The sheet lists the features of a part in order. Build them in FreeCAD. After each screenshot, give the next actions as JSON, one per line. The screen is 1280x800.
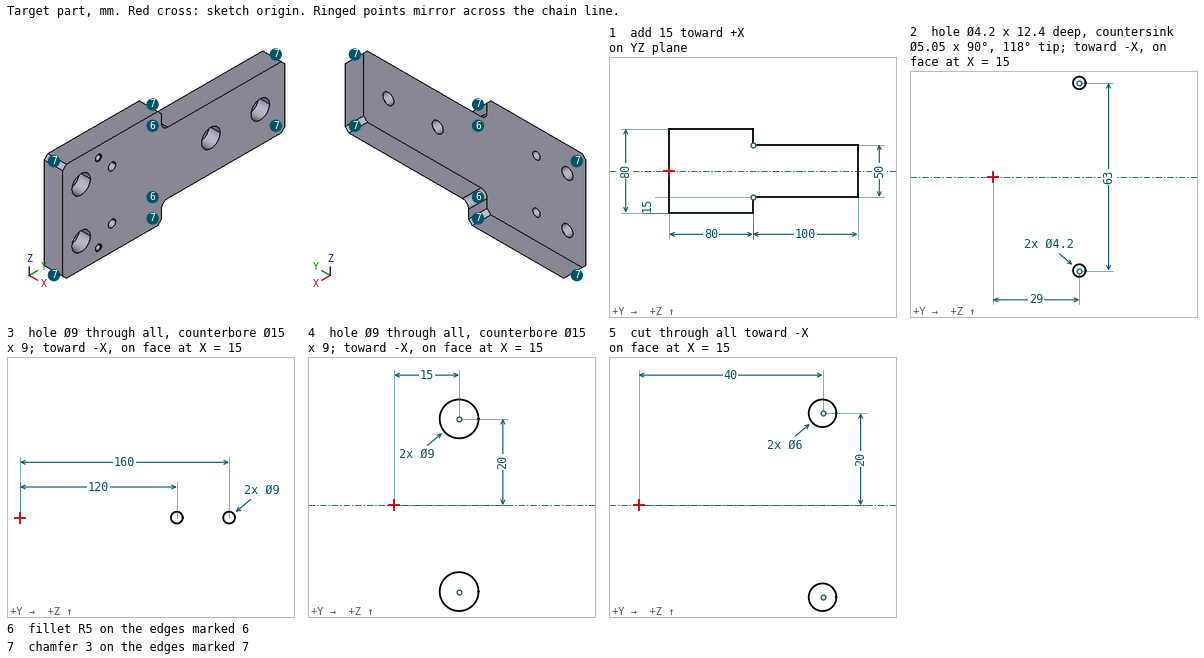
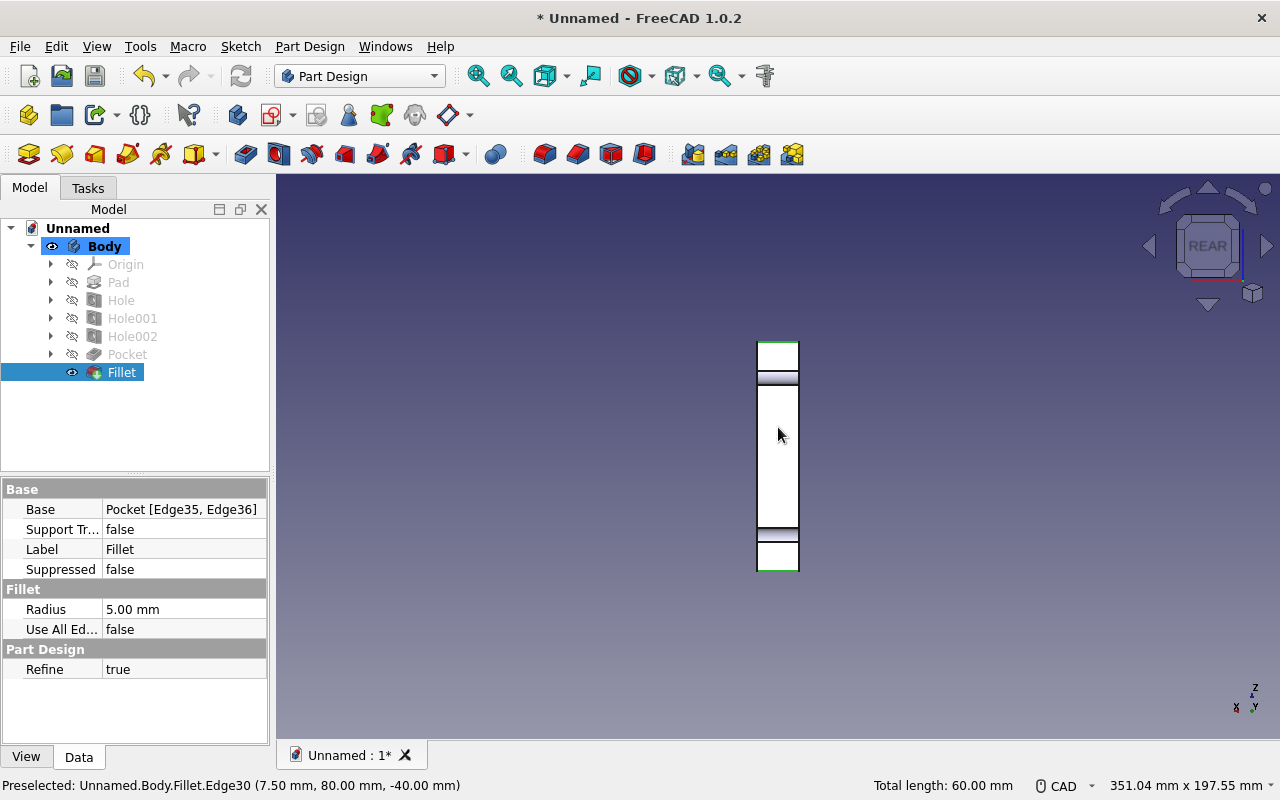
{"action": "left_click", "coordinate": [479, 76]}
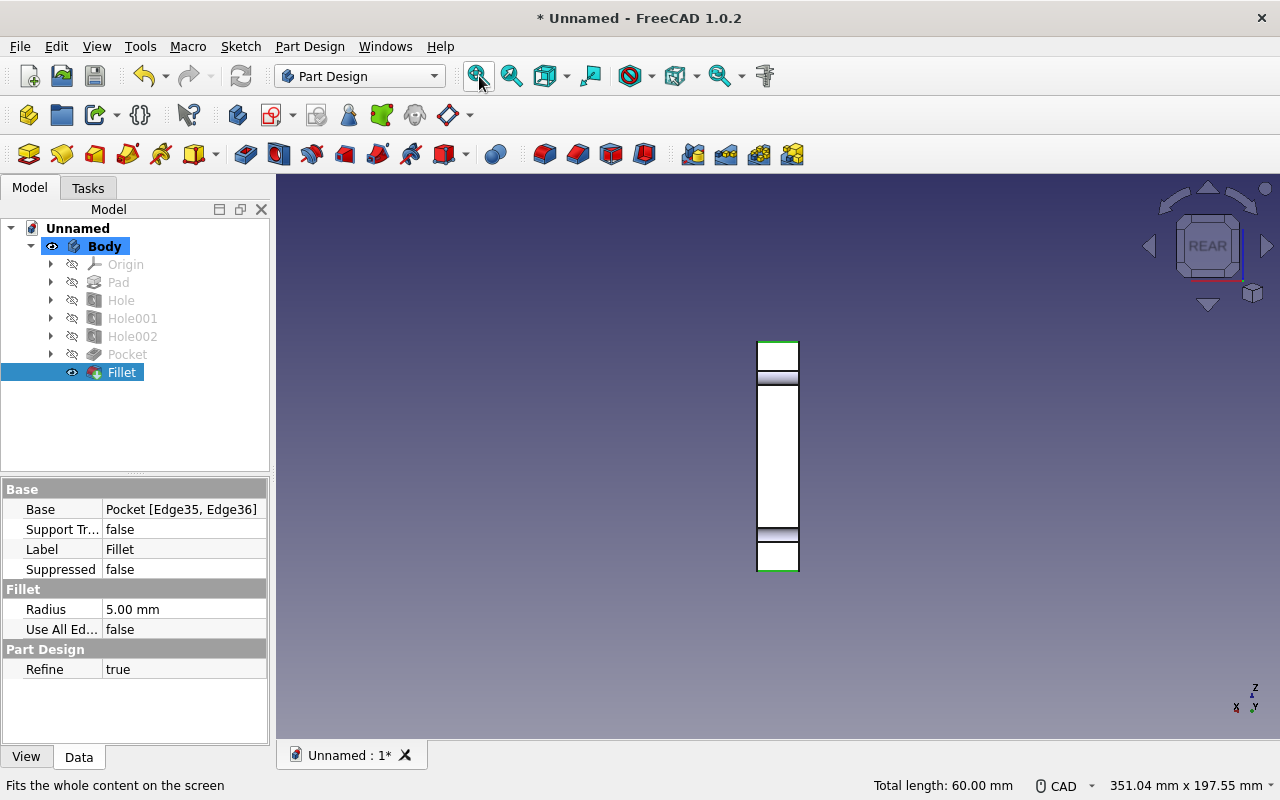
{"action": "left_click", "coordinate": [778, 384], "text": "ctrl"}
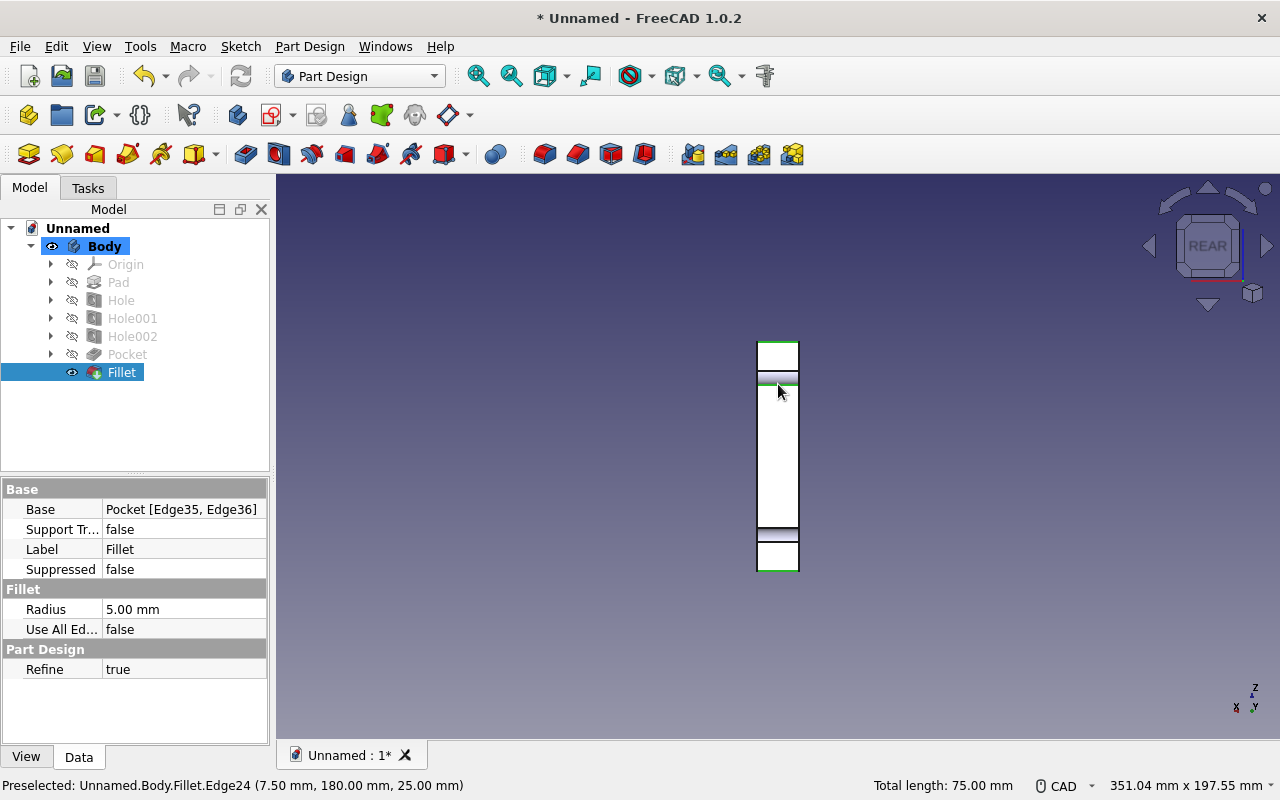
{"action": "left_click", "coordinate": [778, 527], "text": "ctrl"}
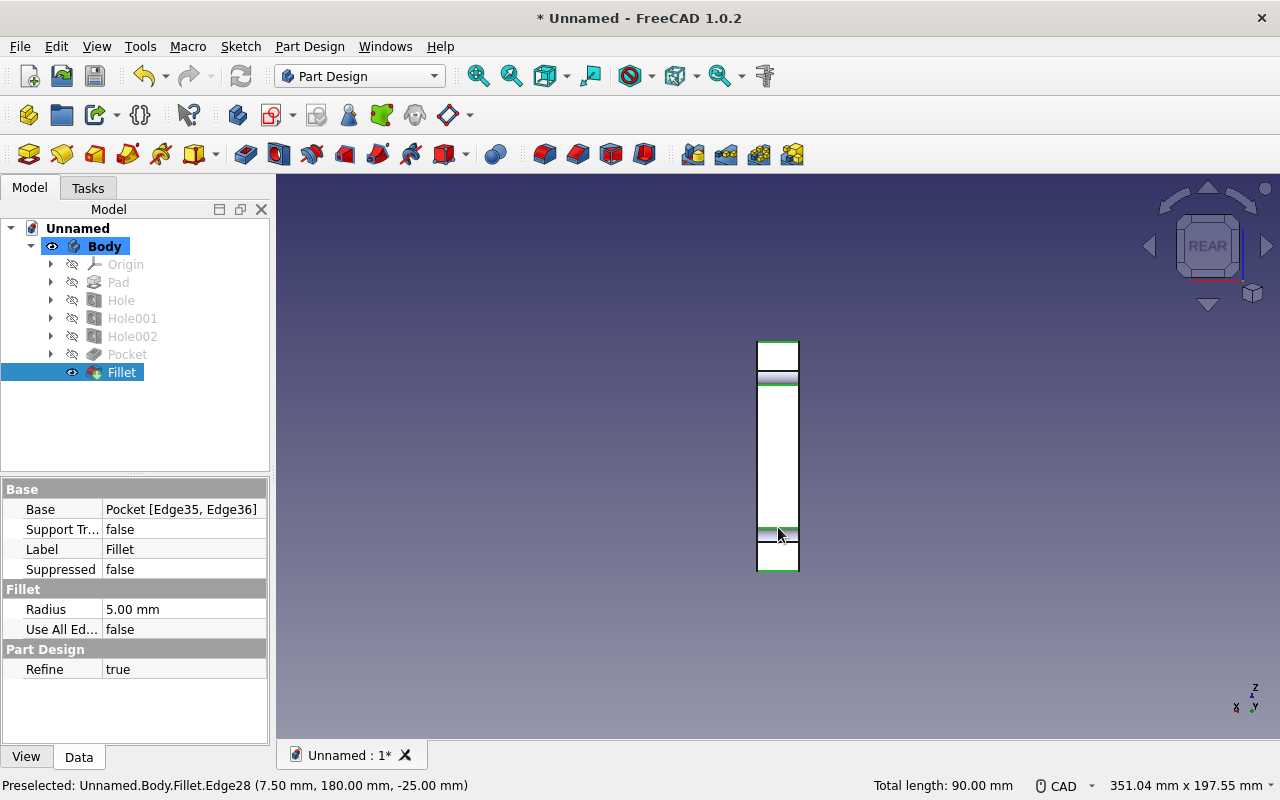
{"action": "left_click", "coordinate": [578, 154]}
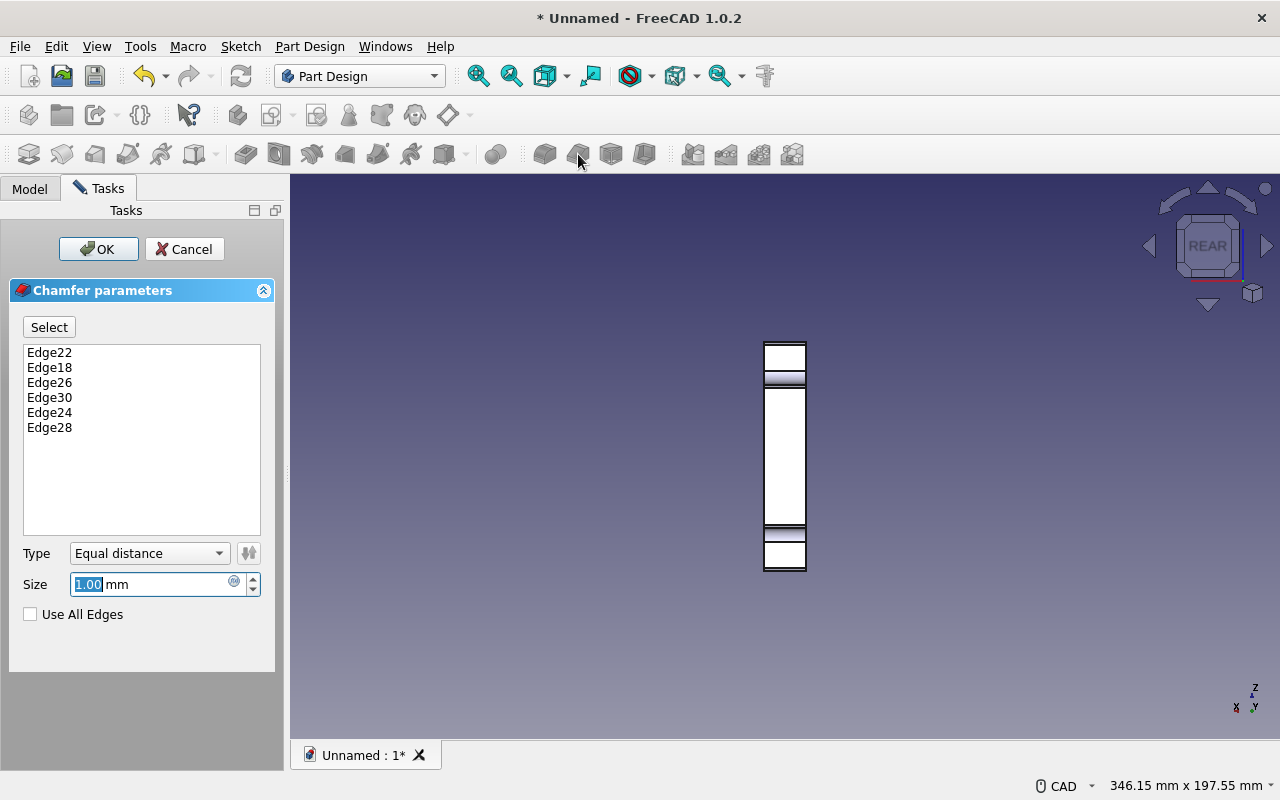
{"action": "type", "text": "3"}
{"action": "key", "text": "Tab"}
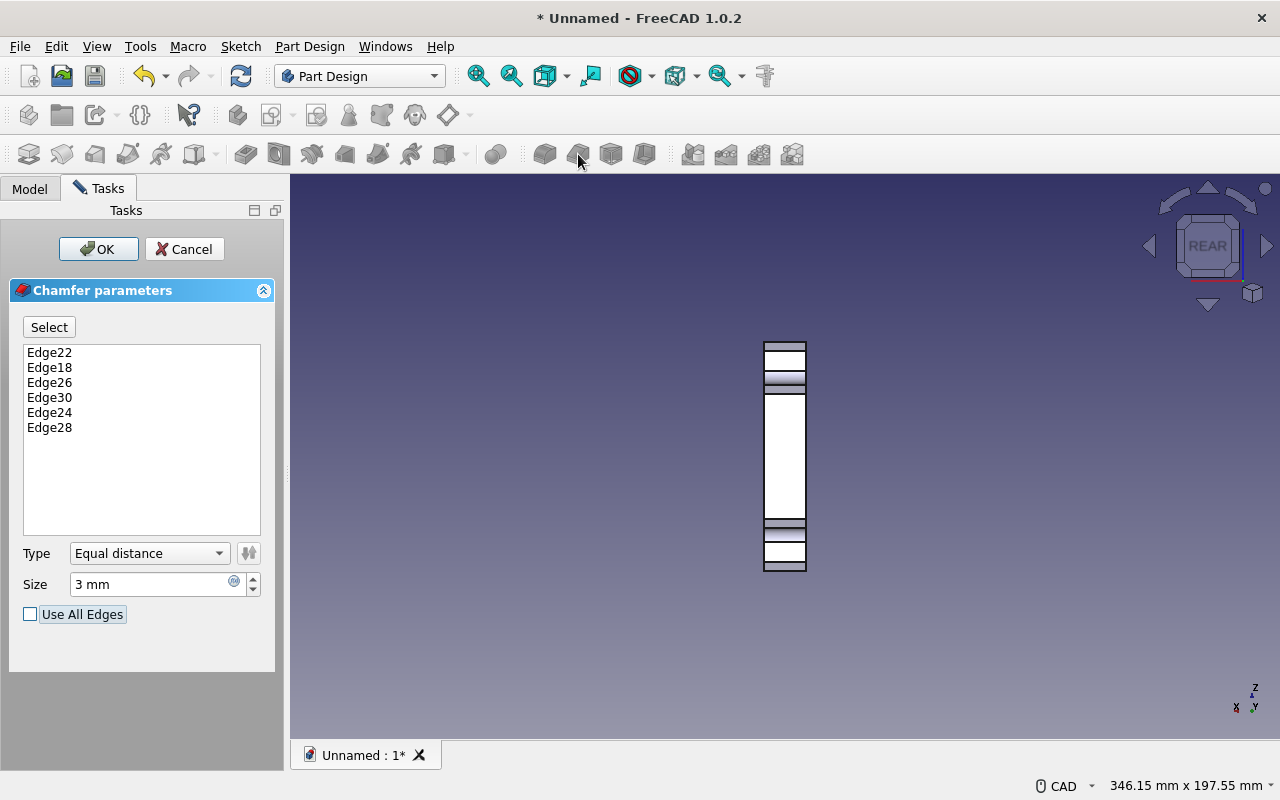
{"action": "left_click", "coordinate": [99, 249]}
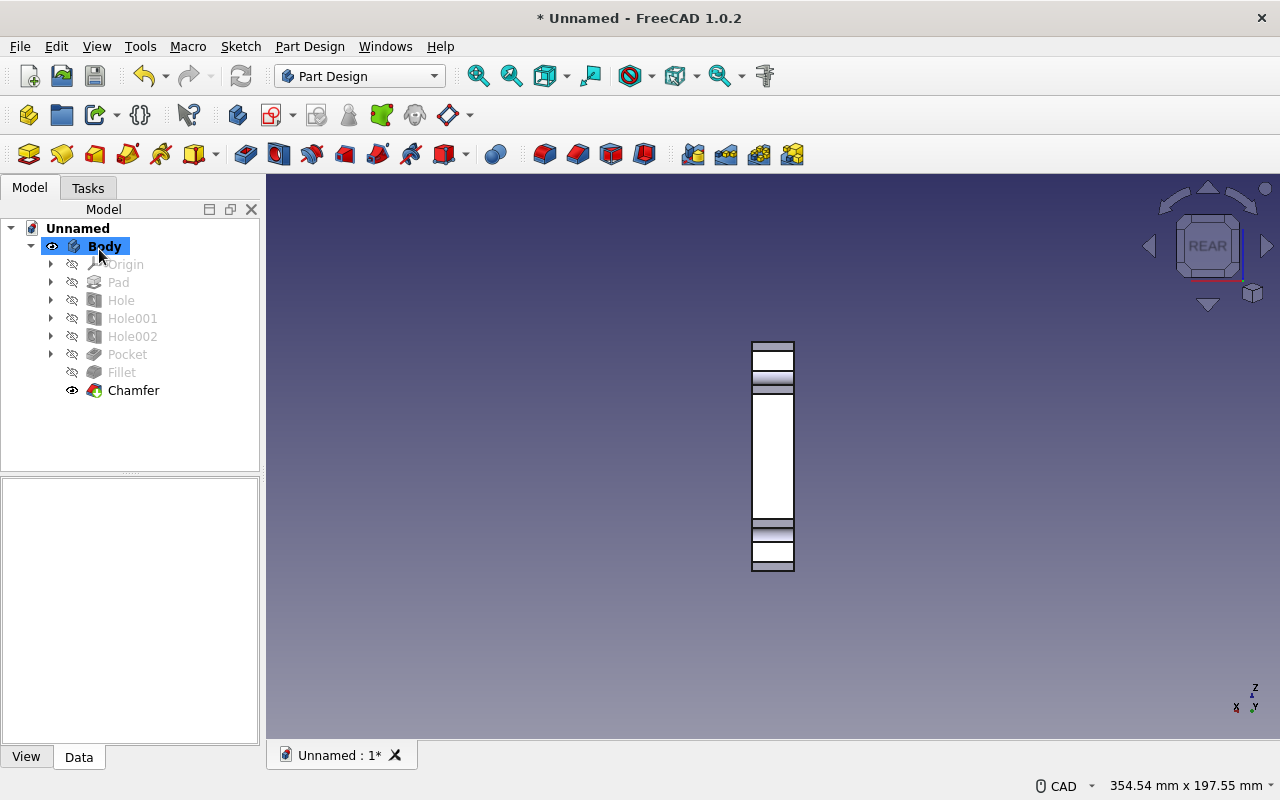
{"action": "key", "text": "0"}